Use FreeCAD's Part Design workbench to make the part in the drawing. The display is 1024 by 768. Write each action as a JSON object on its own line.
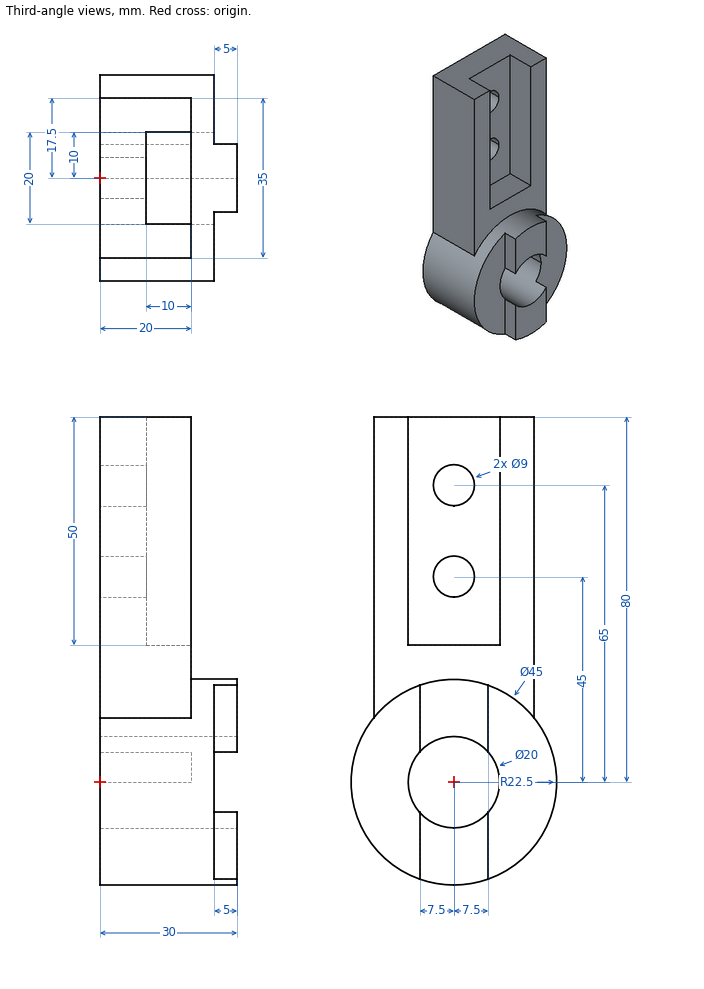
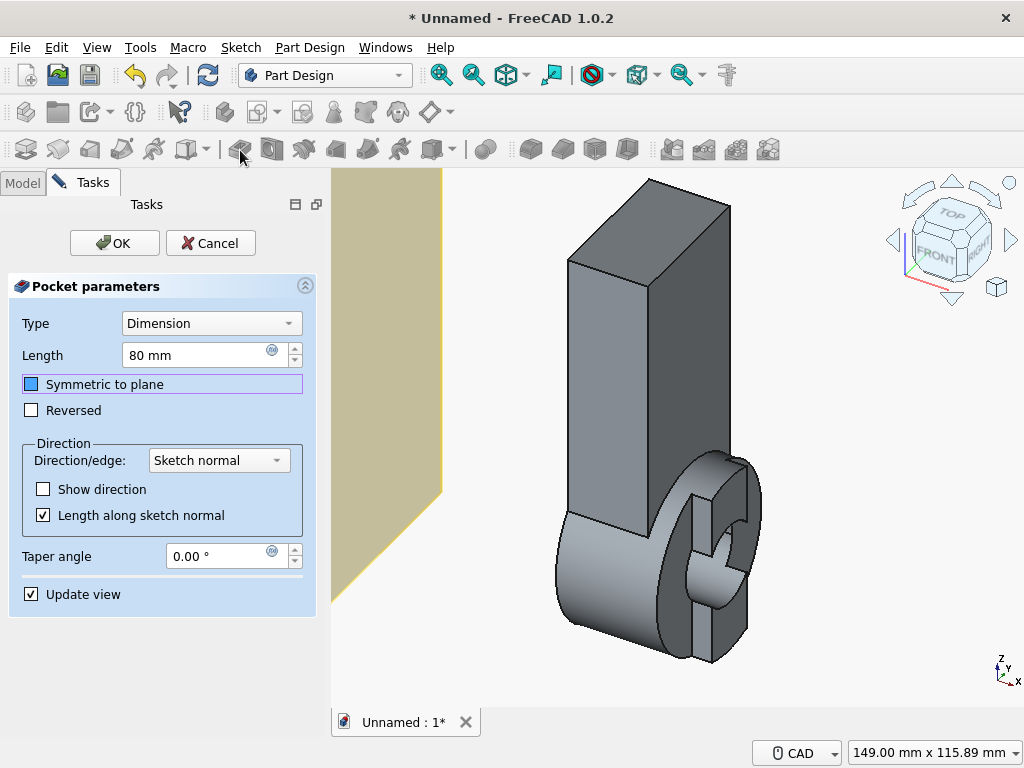
{"action": "left_click", "coordinate": [30, 410]}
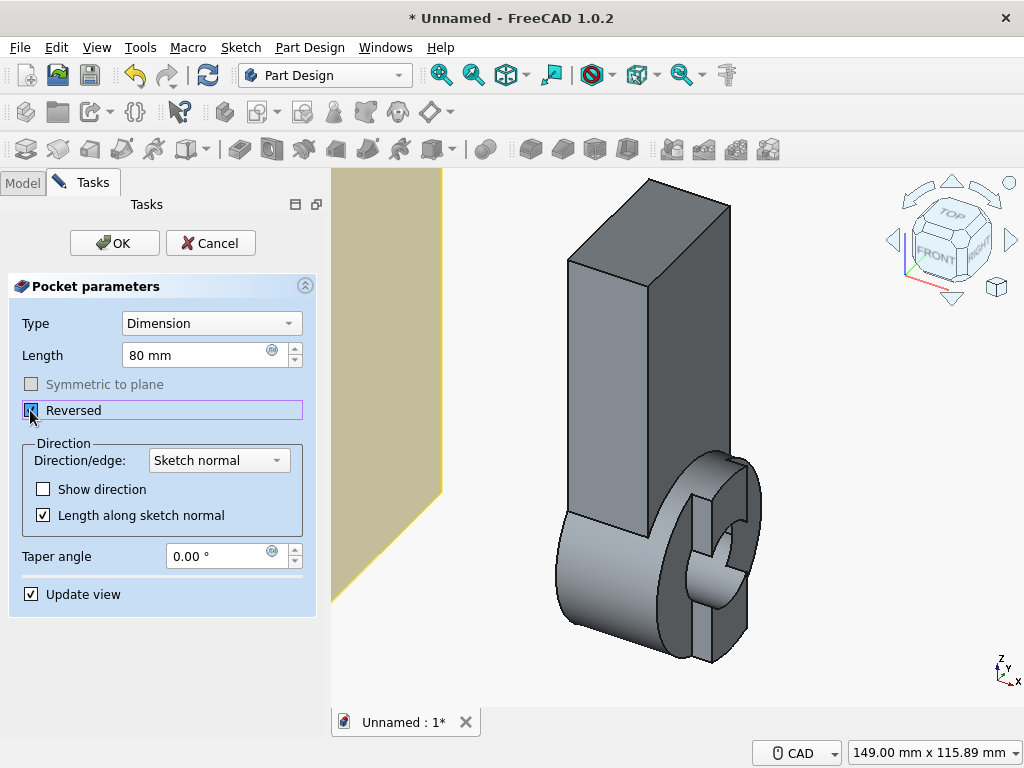
{"action": "left_click", "coordinate": [115, 243]}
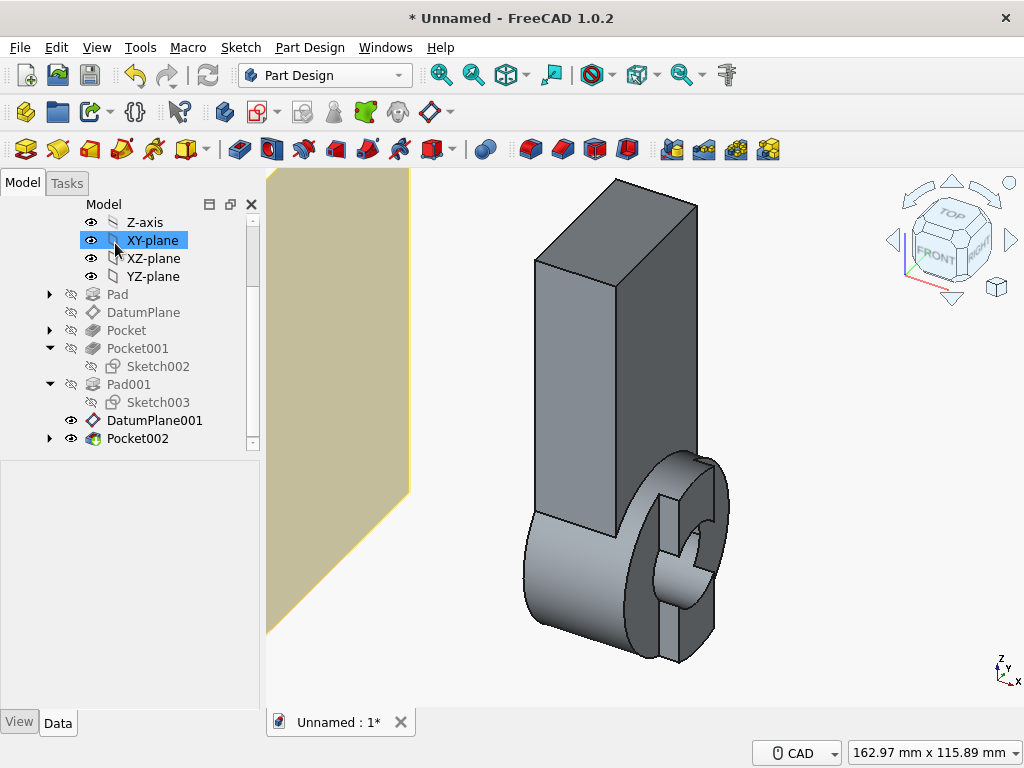
{"action": "left_click", "coordinate": [116, 420]}
{"action": "key", "text": "space"}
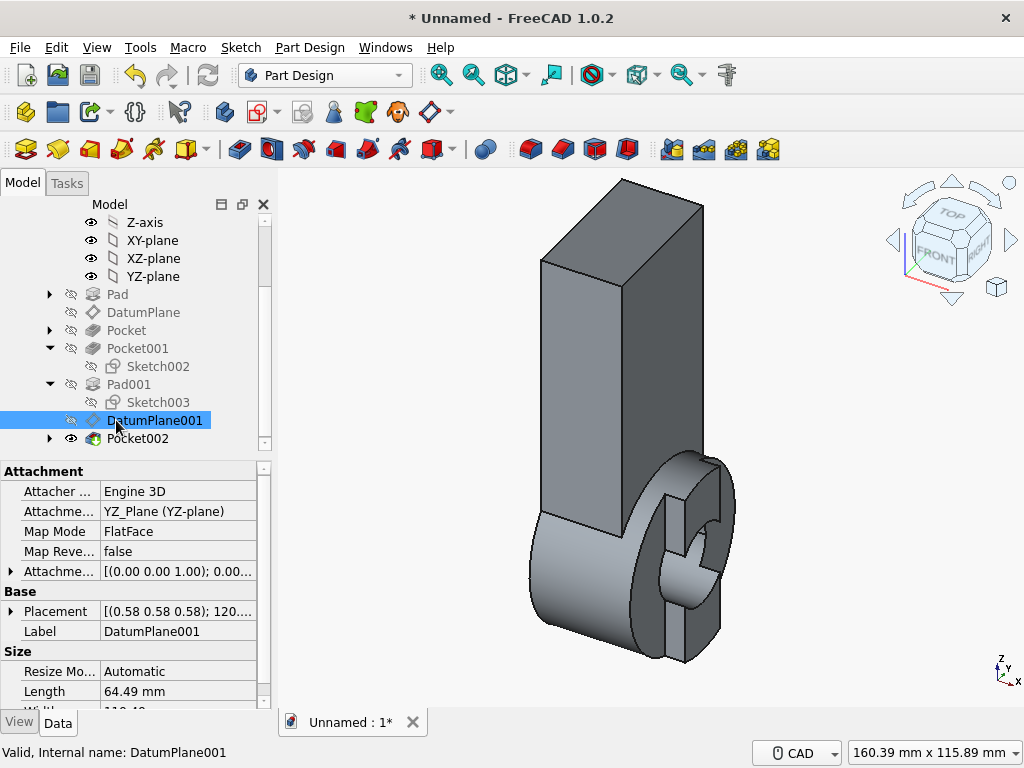
{"action": "left_click", "coordinate": [442, 76]}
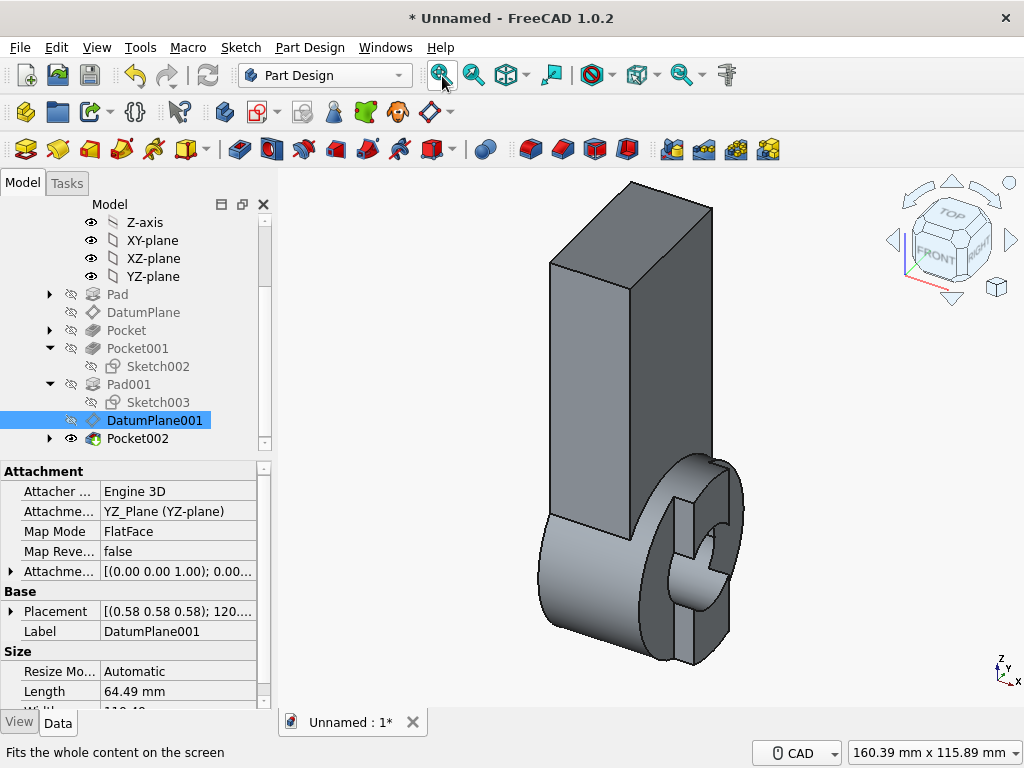
{"action": "left_click", "coordinate": [642, 223]}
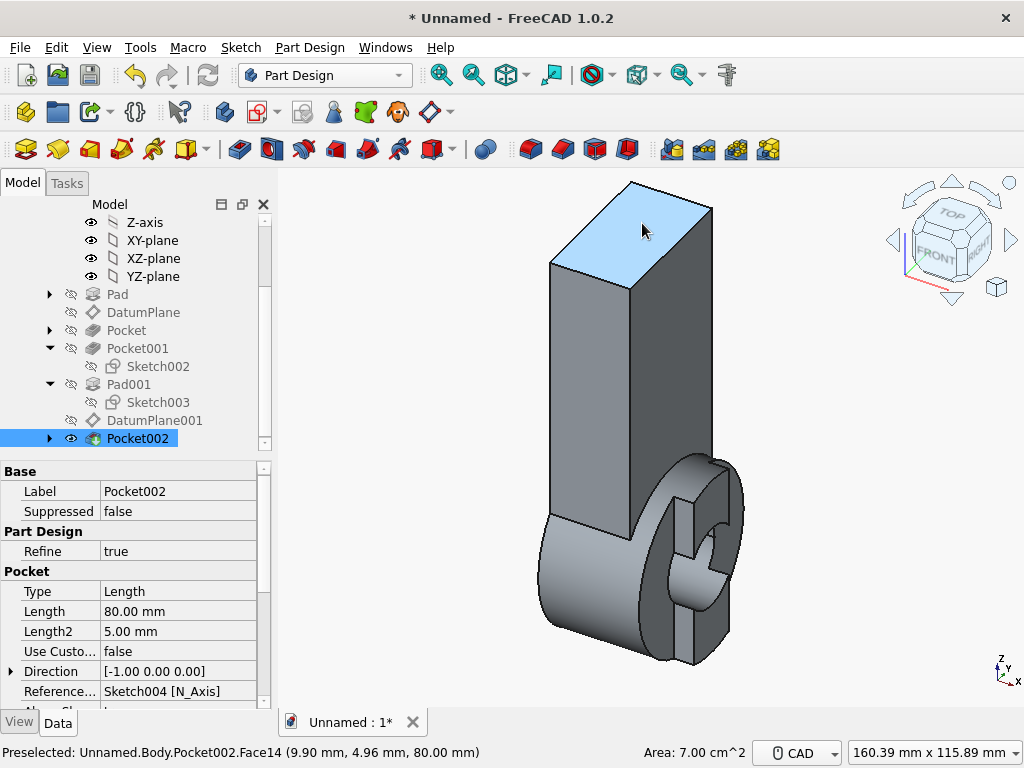
{"action": "left_click", "coordinate": [258, 112]}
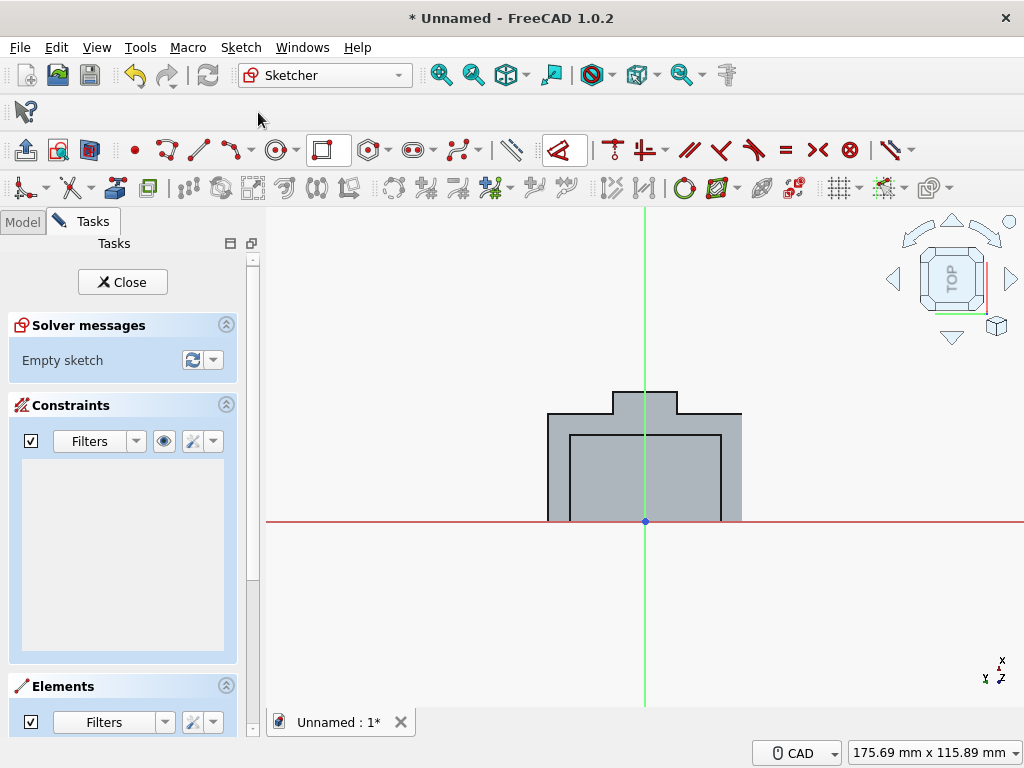
{"action": "scroll", "coordinate": [675, 488], "scroll_direction": "up", "scroll_amount": 6}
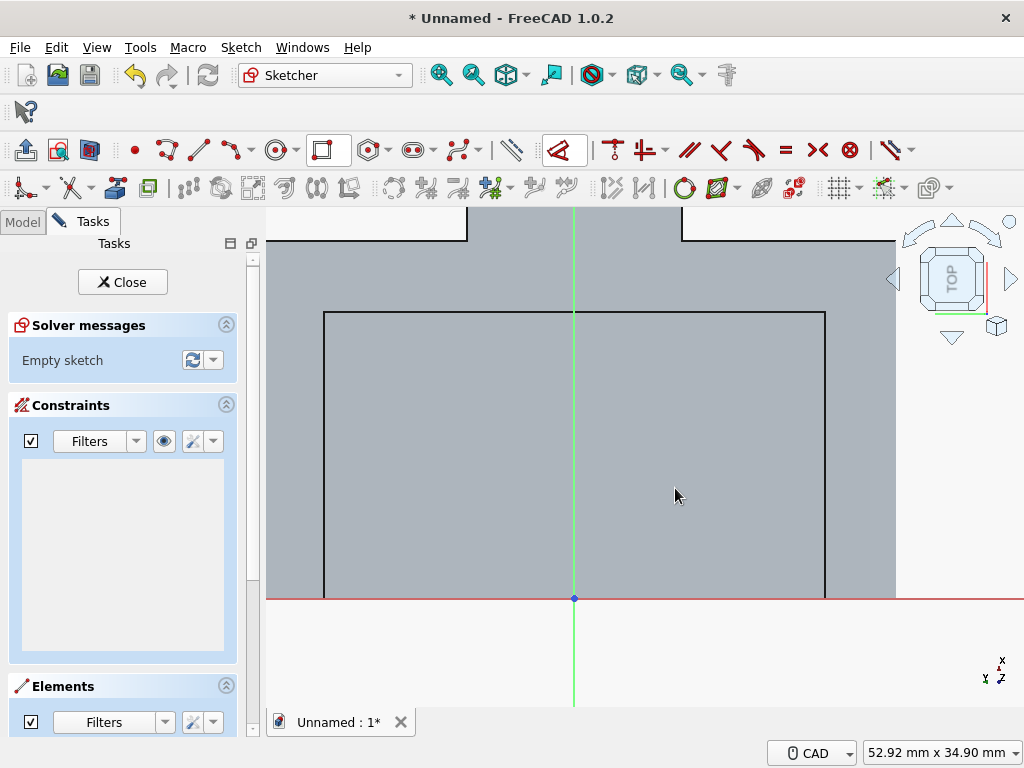
{"action": "left_click", "coordinate": [322, 150]}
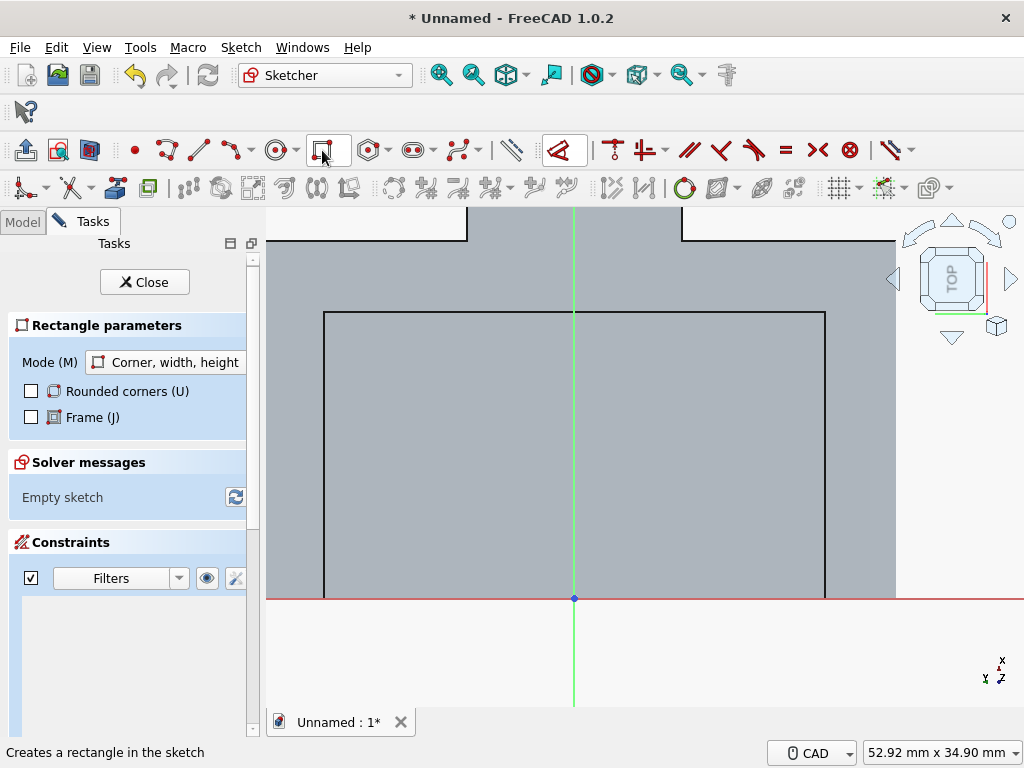
{"action": "left_click", "coordinate": [431, 312]}
{"action": "mouse_move", "coordinate": [717, 455]}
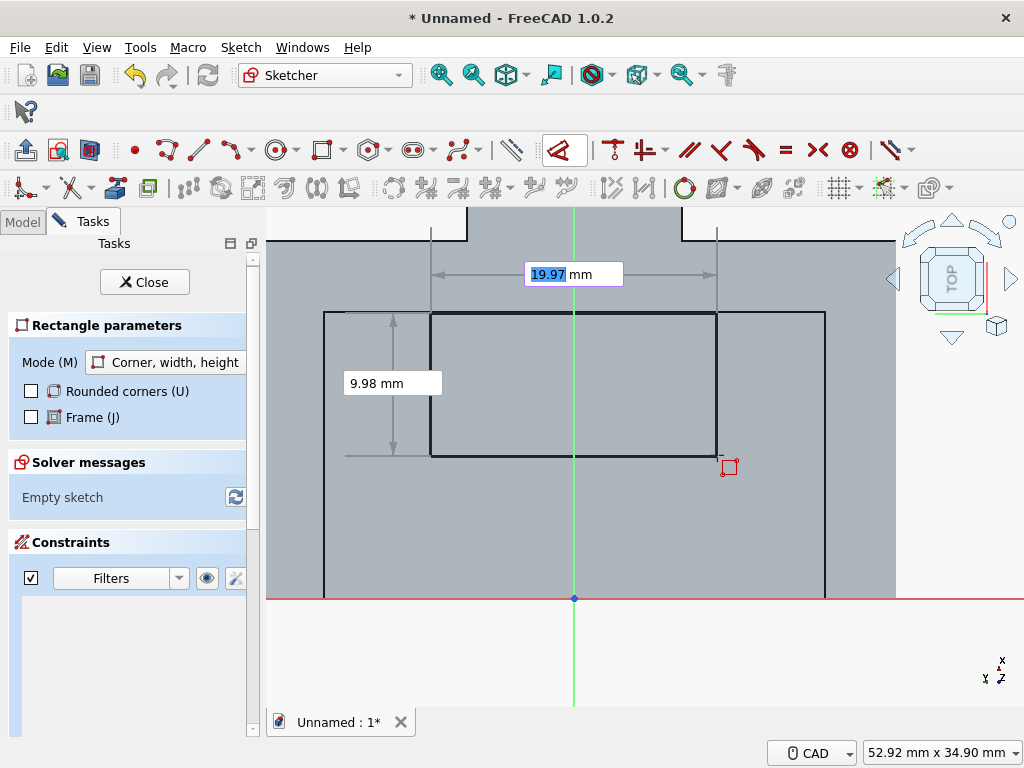
{"action": "type", "text": "20"}
{"action": "key", "text": "Tab"}
{"action": "type", "text": "10"}
{"action": "key", "text": "Return"}
{"action": "key", "text": "Escape"}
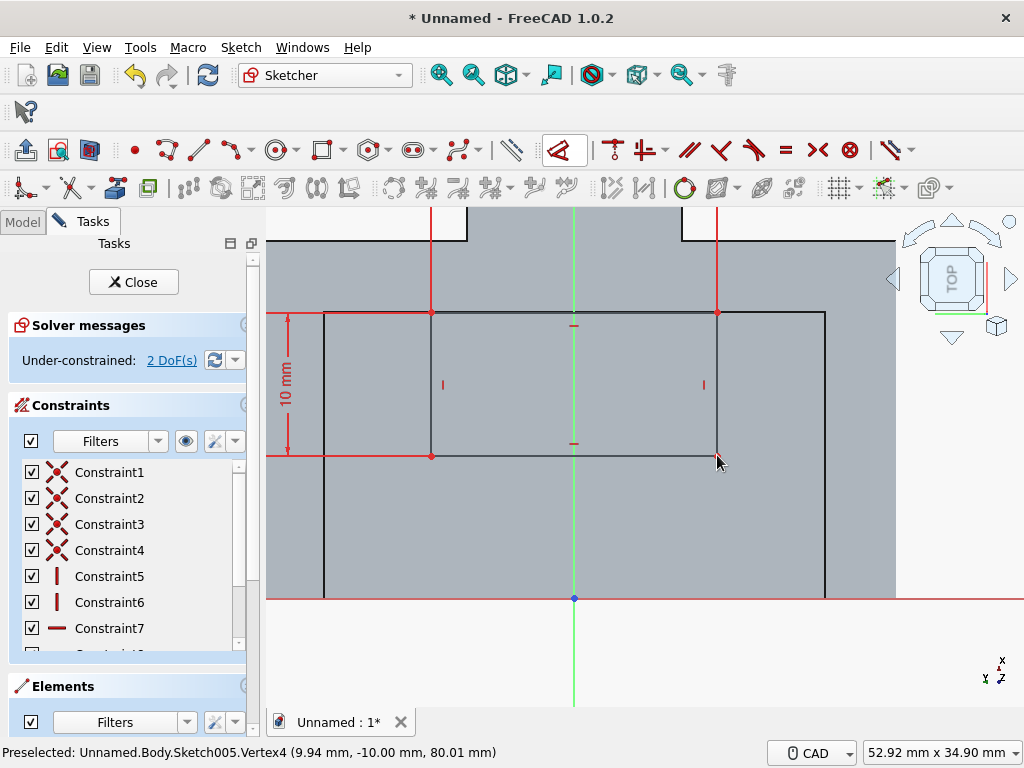
{"action": "left_click", "coordinate": [431, 313]}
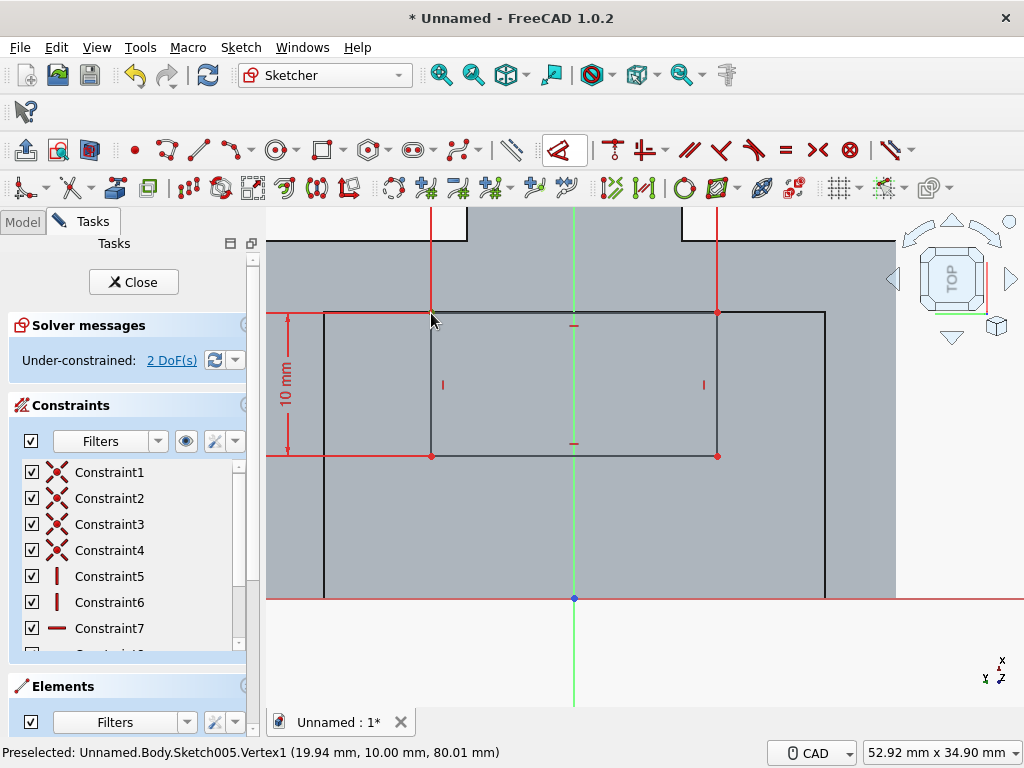
{"action": "key", "text": "l"}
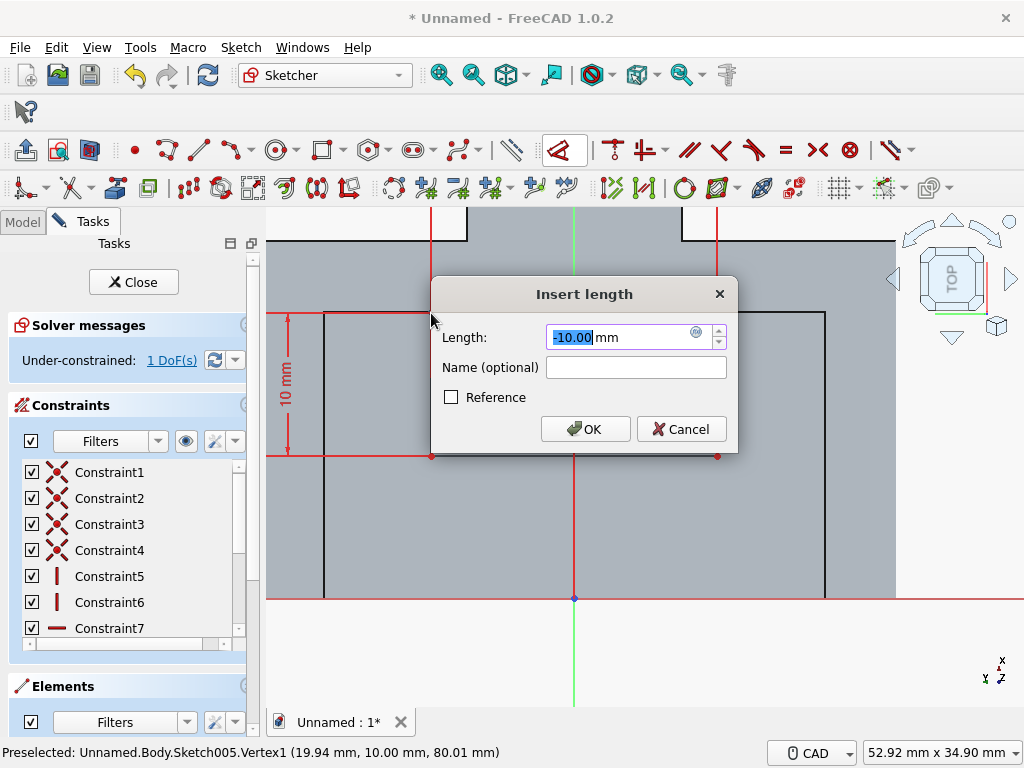
{"action": "type", "text": "-10"}
{"action": "key", "text": "Return"}